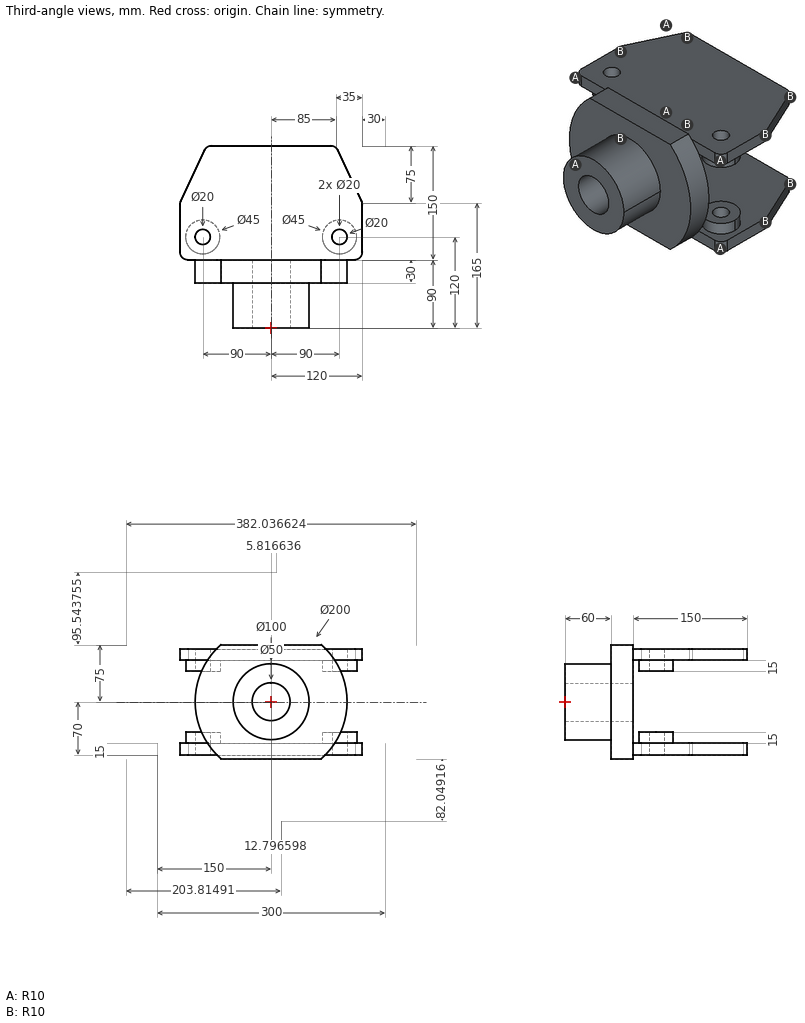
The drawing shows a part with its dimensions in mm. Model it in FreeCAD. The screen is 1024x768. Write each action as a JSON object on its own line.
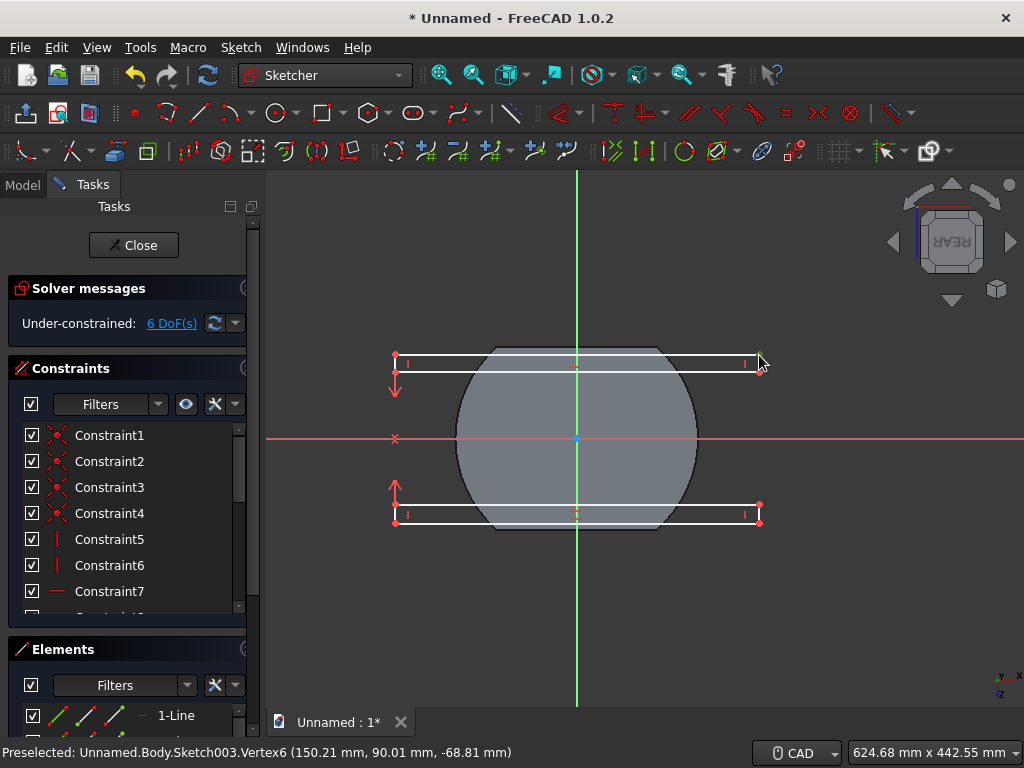
{"action": "left_click", "coordinate": [759, 524]}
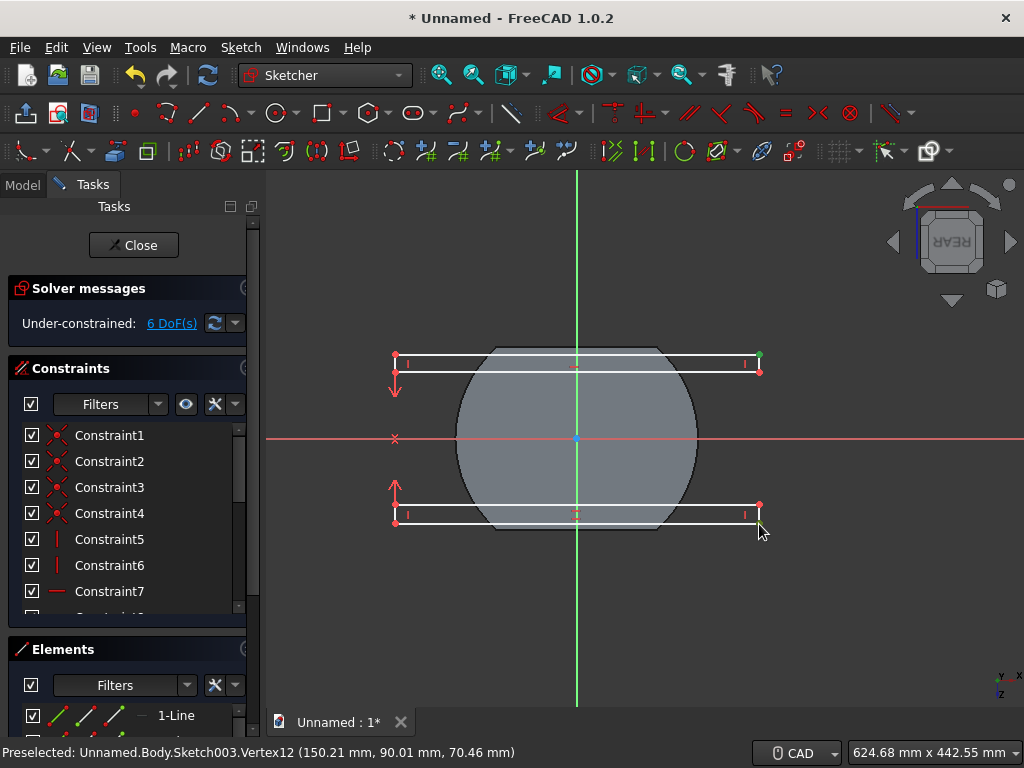
{"action": "left_click", "coordinate": [334, 439]}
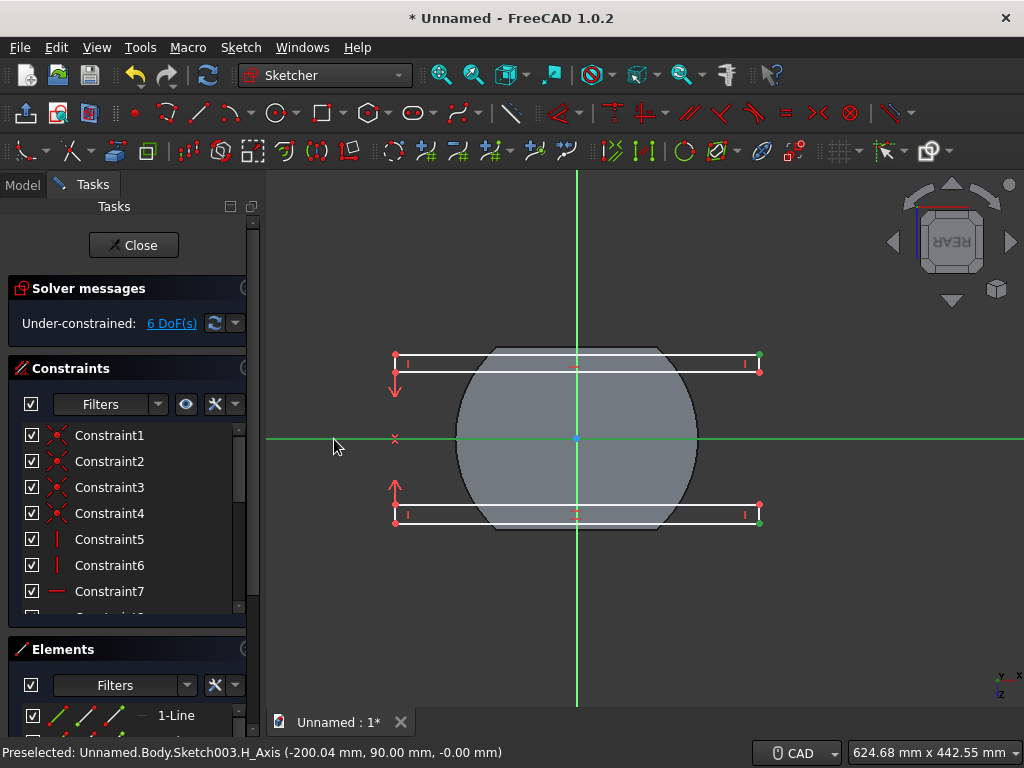
{"action": "left_click", "coordinate": [818, 114]}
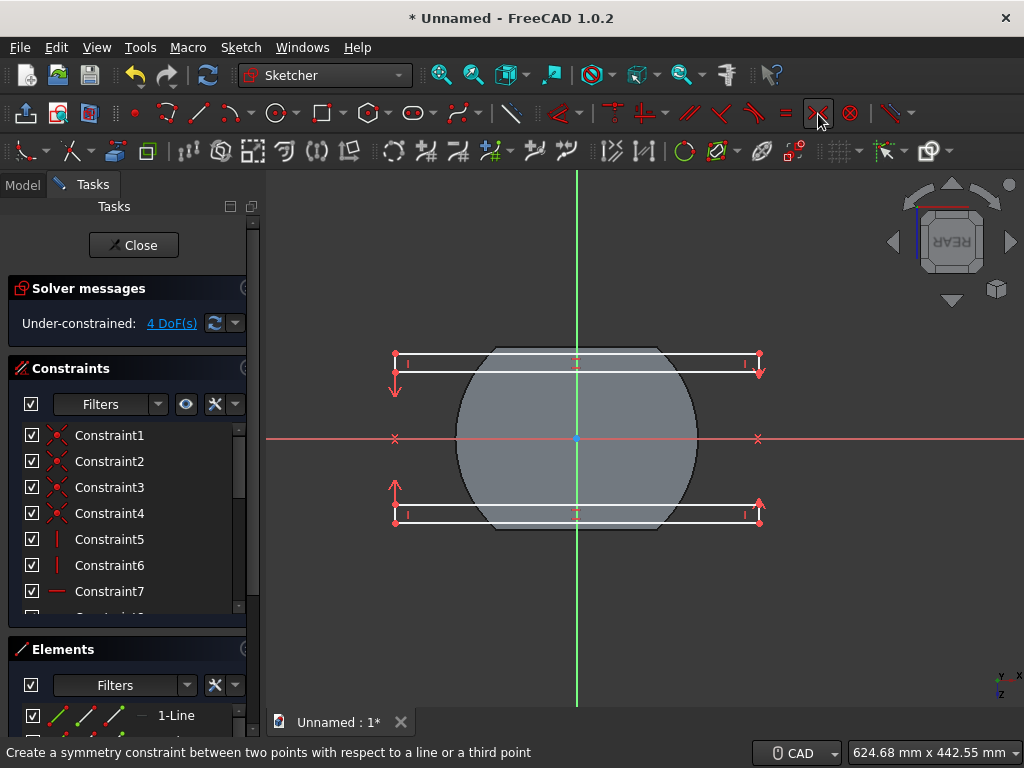
{"action": "left_click", "coordinate": [558, 114]}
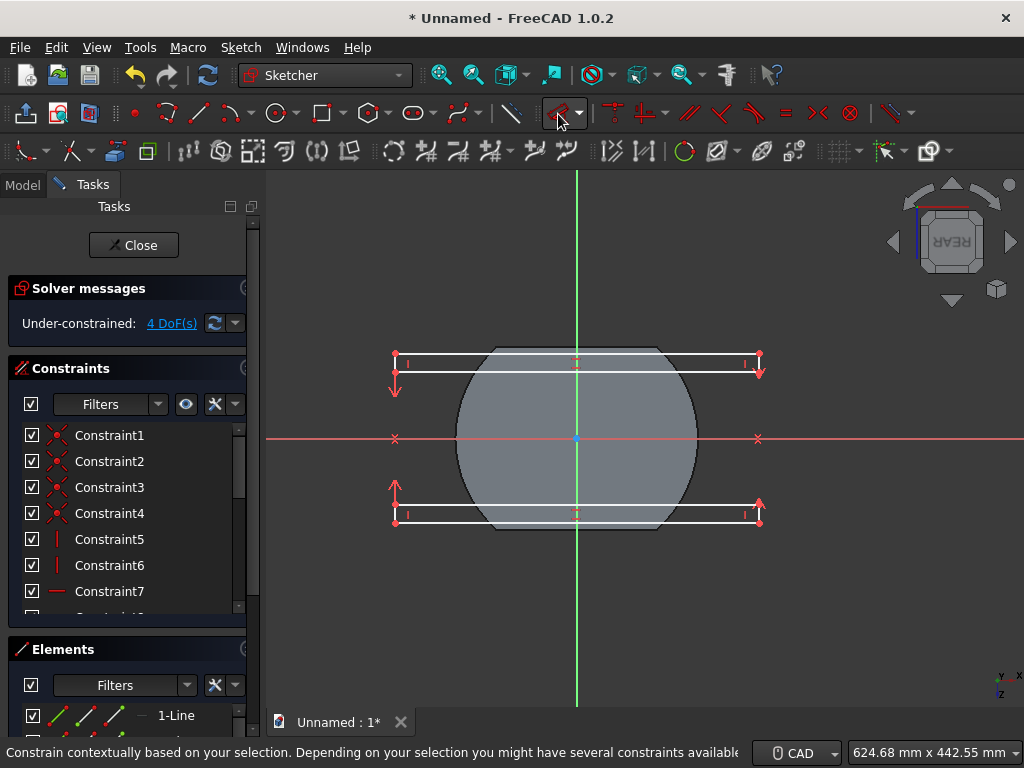
{"action": "scroll", "coordinate": [395, 363], "scroll_direction": "up", "scroll_amount": 4}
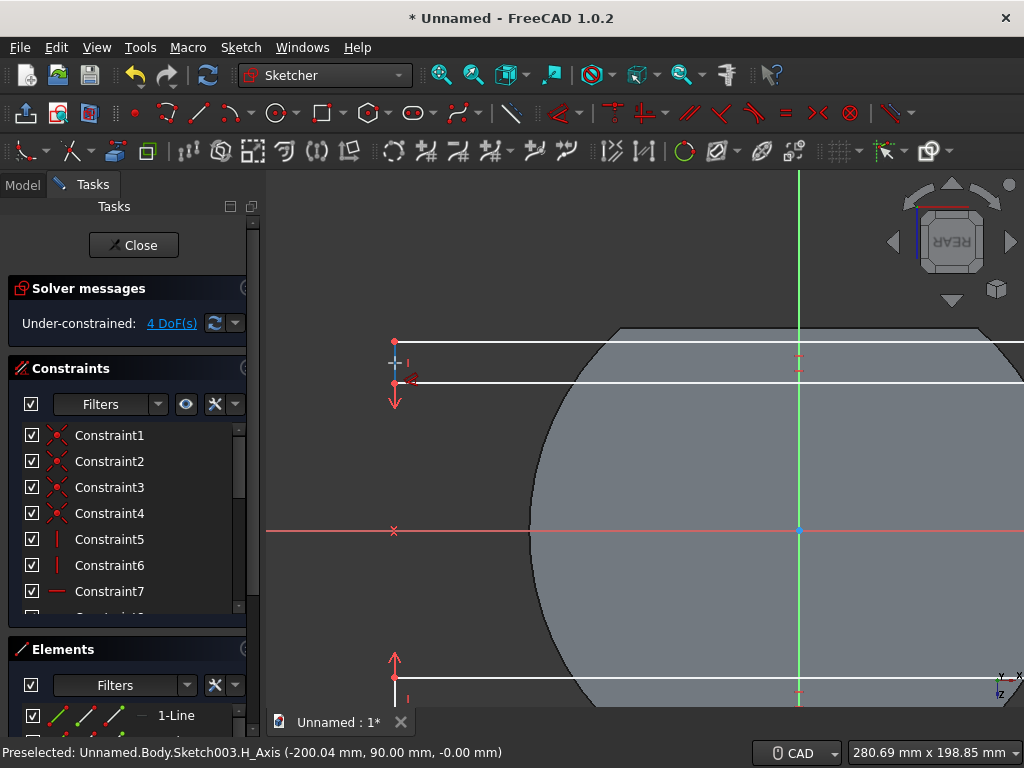
{"action": "left_click", "coordinate": [395, 363]}
{"action": "left_click", "coordinate": [361, 363]}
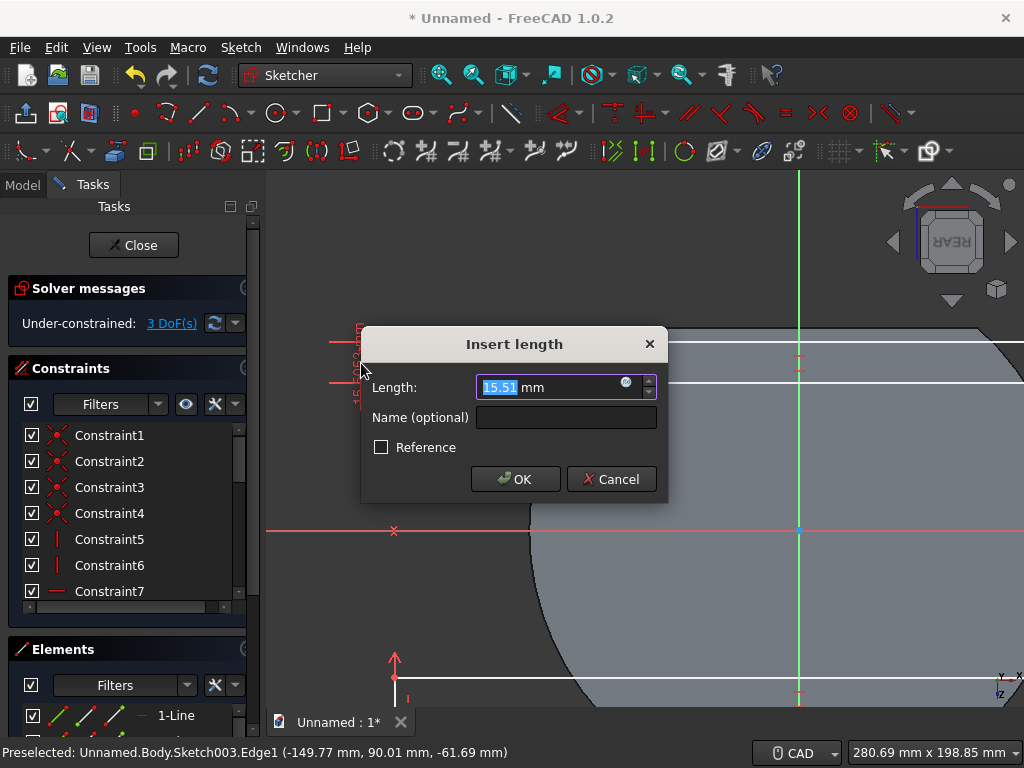
{"action": "type", "text": "15"}
{"action": "key", "text": "Return"}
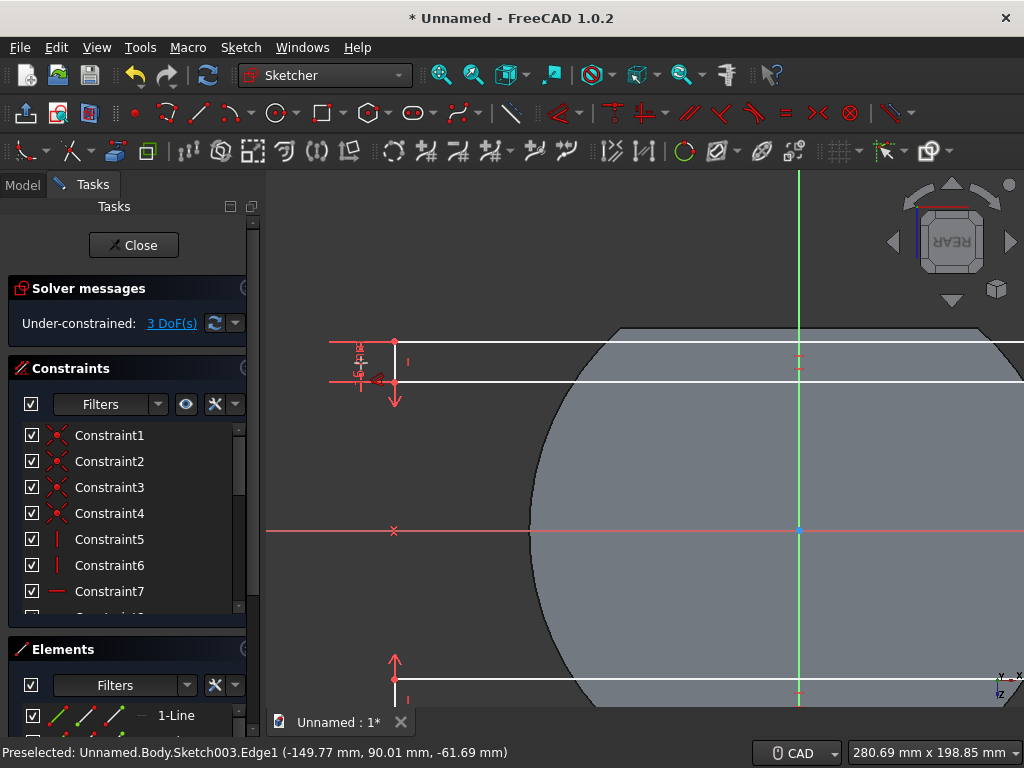
{"action": "left_click", "coordinate": [638, 382]}
{"action": "left_click", "coordinate": [627, 416]}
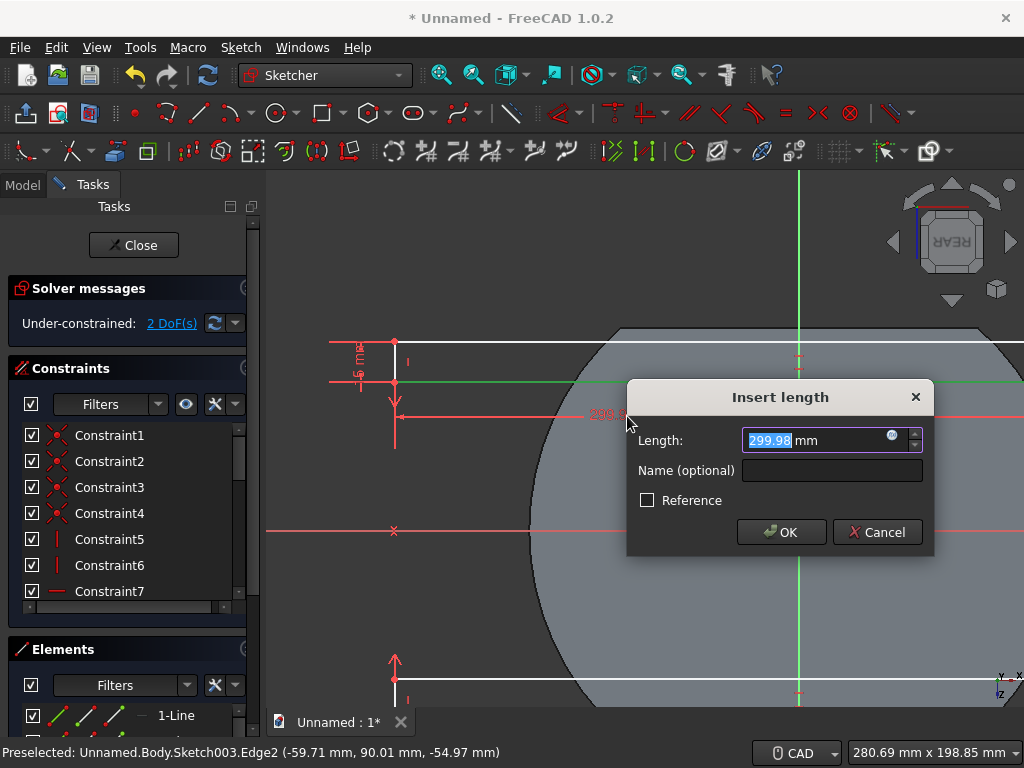
{"action": "type", "text": "300"}
{"action": "key", "text": "Return"}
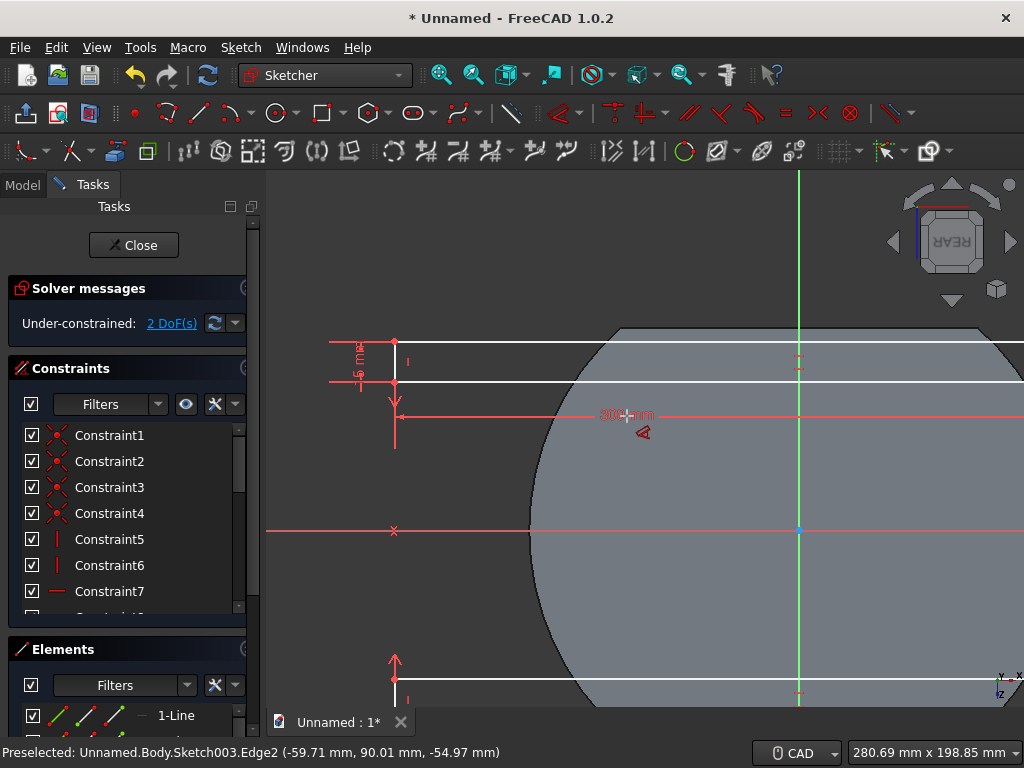
{"action": "left_click", "coordinate": [395, 342]}
{"action": "left_click", "coordinate": [361, 436]}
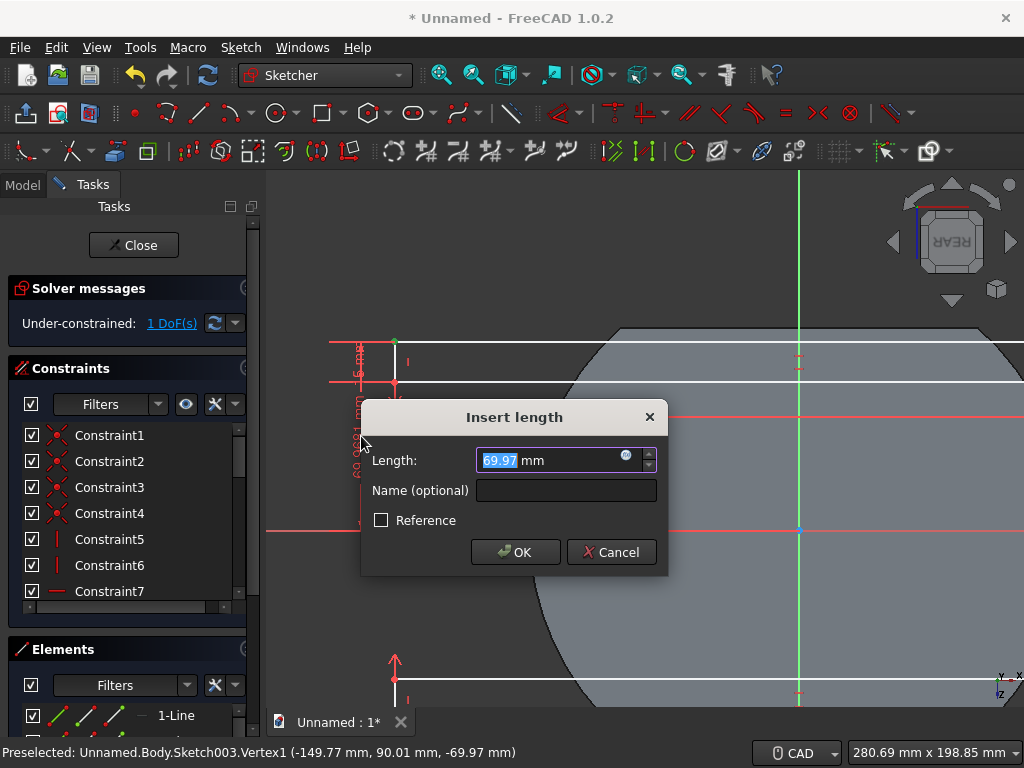
{"action": "type", "text": "70"}
{"action": "key", "text": "Return"}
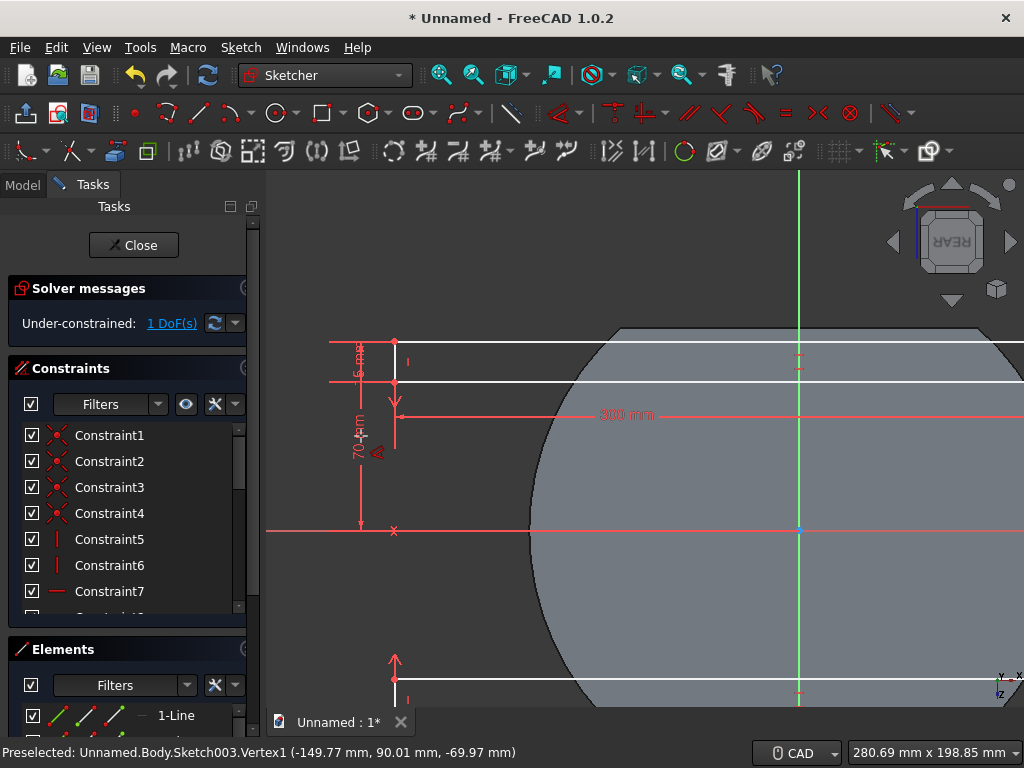
{"action": "left_click", "coordinate": [395, 342]}
{"action": "left_click", "coordinate": [597, 308]}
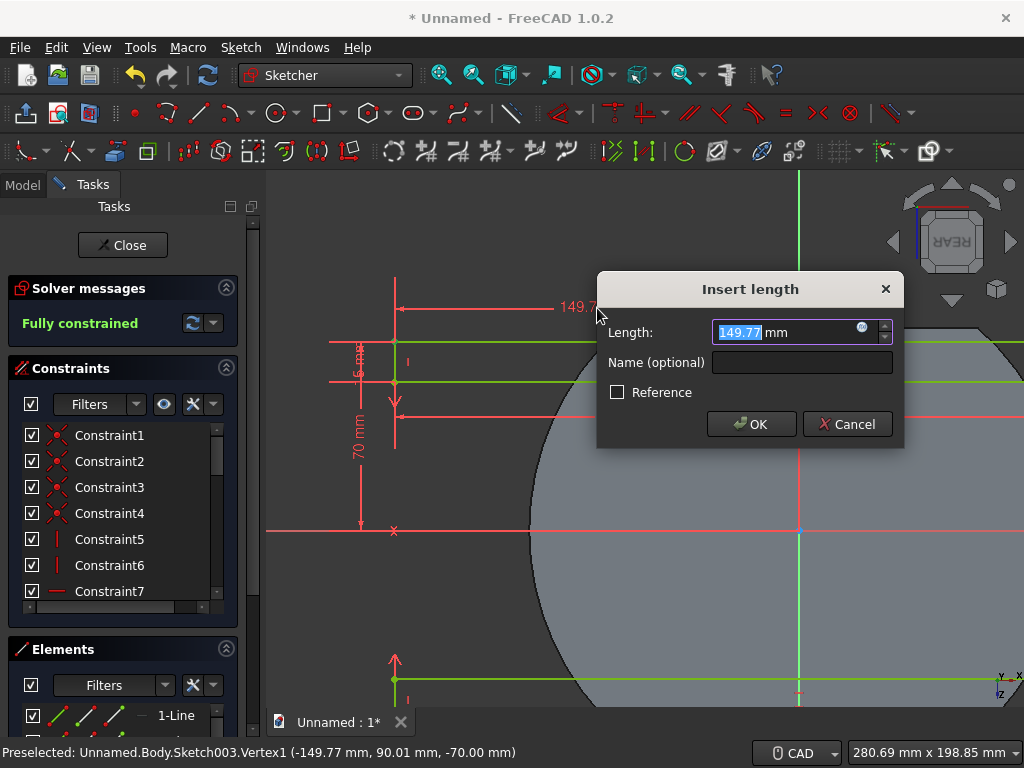
{"action": "type", "text": "150"}
{"action": "key", "text": "Return"}
{"action": "key", "text": "Escape"}